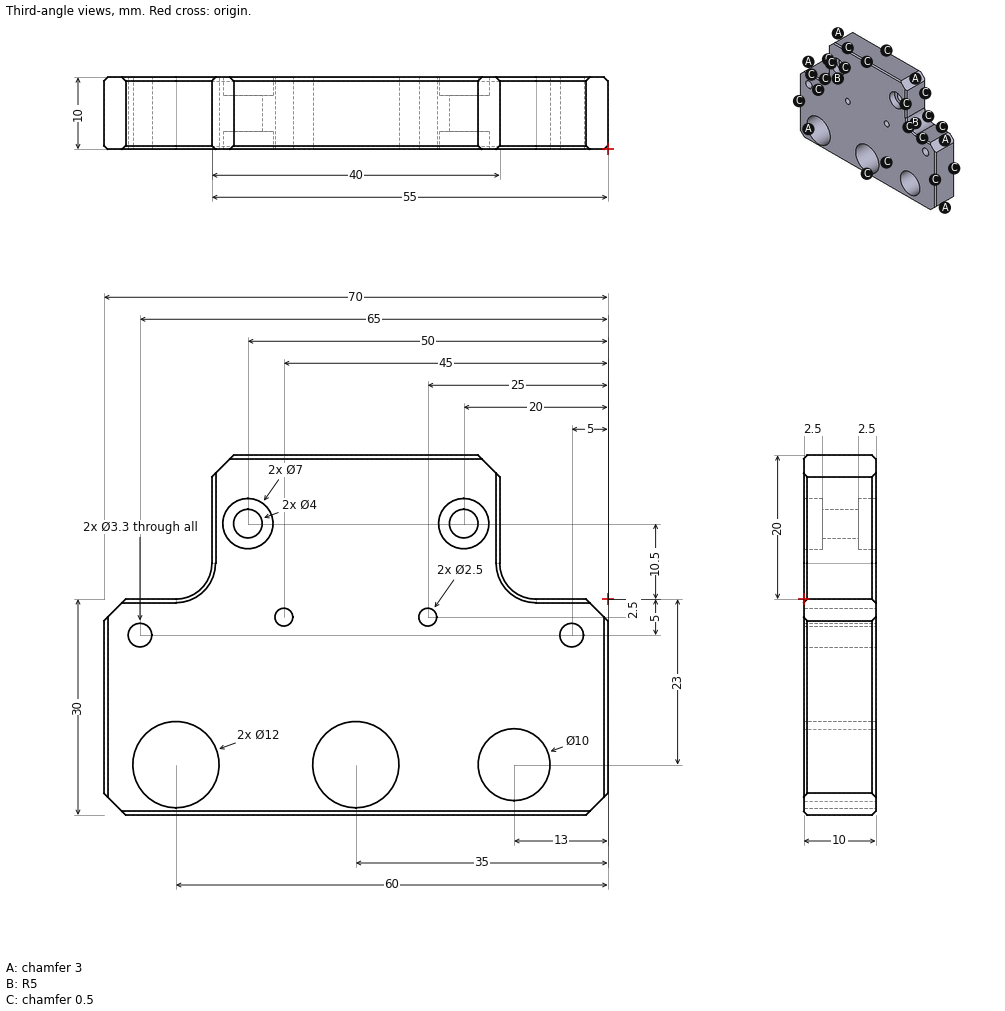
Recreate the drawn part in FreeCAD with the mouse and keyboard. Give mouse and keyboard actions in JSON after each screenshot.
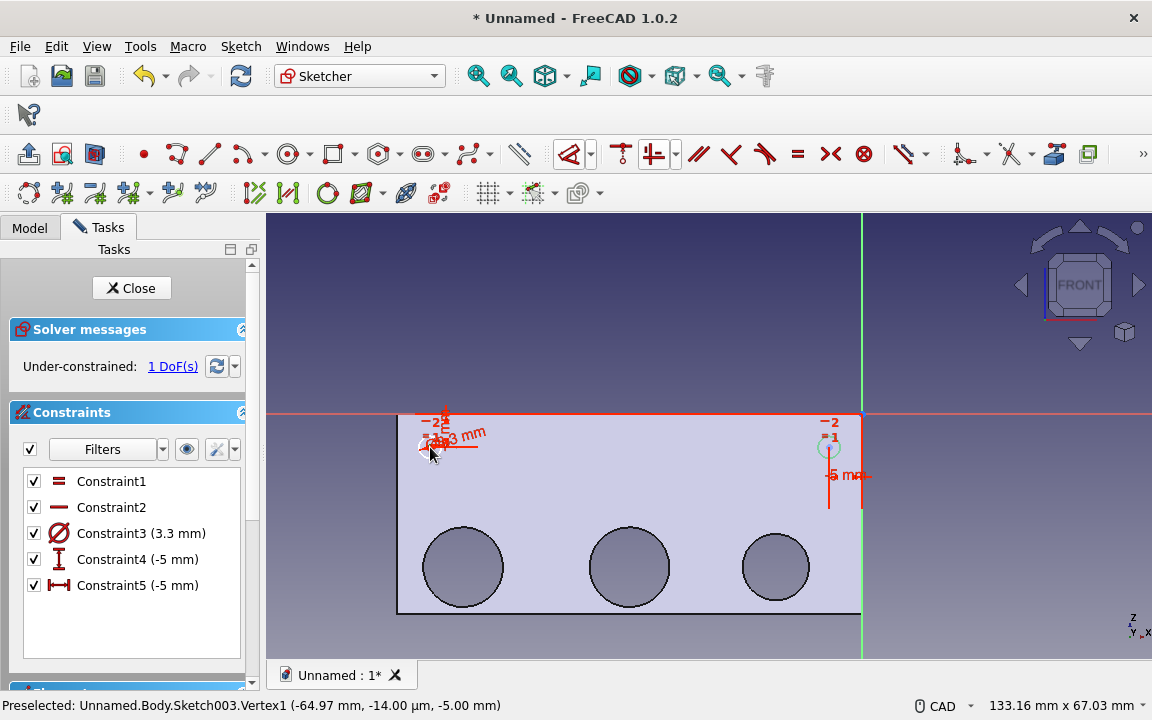
{"action": "left_click", "coordinate": [590, 154]}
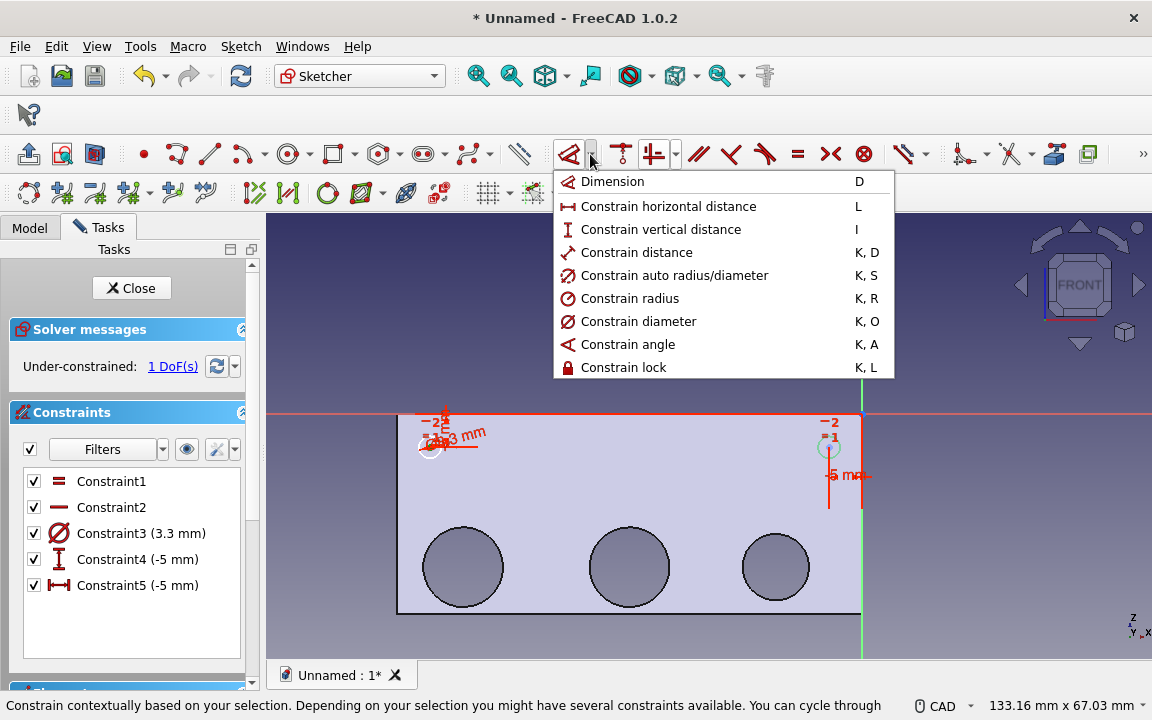
{"action": "left_click", "coordinate": [724, 206]}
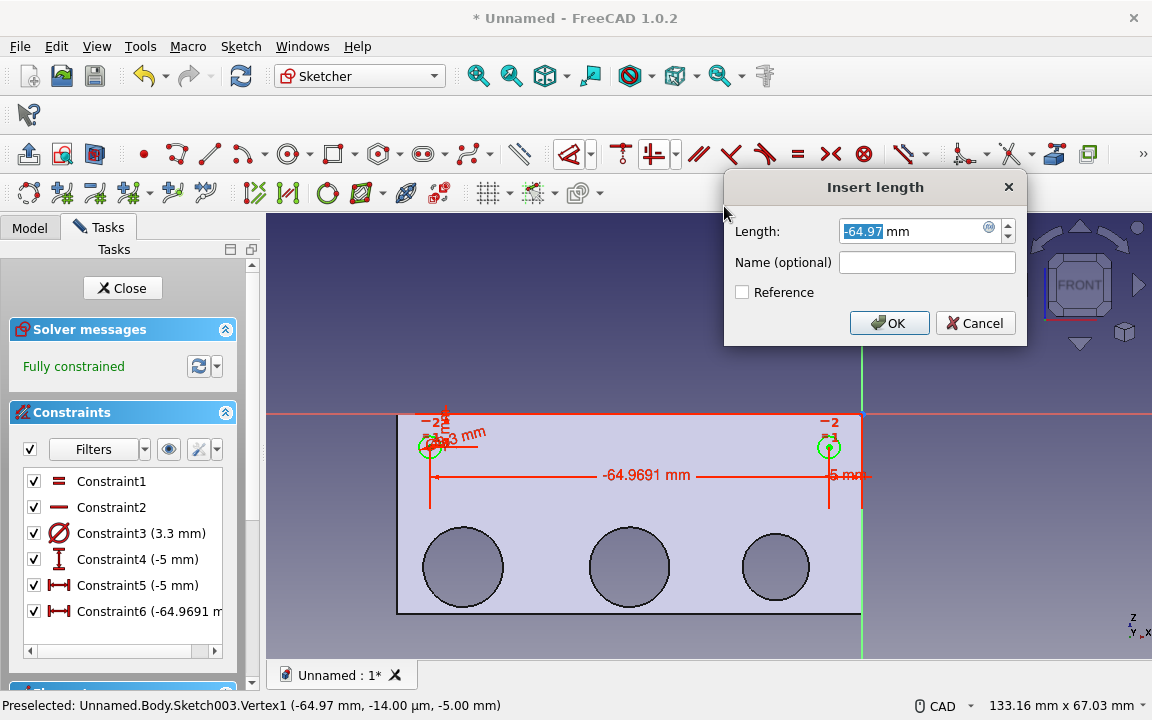
{"action": "type", "text": "-65"}
{"action": "key", "text": "Return"}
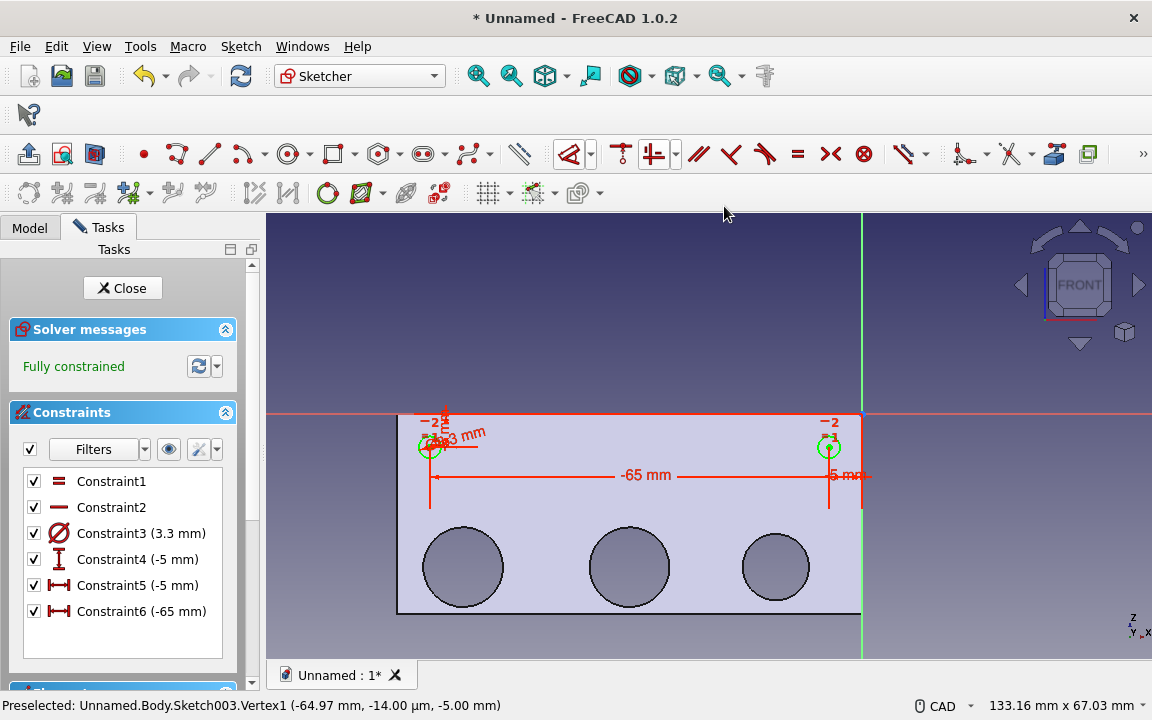
{"action": "left_click", "coordinate": [123, 288]}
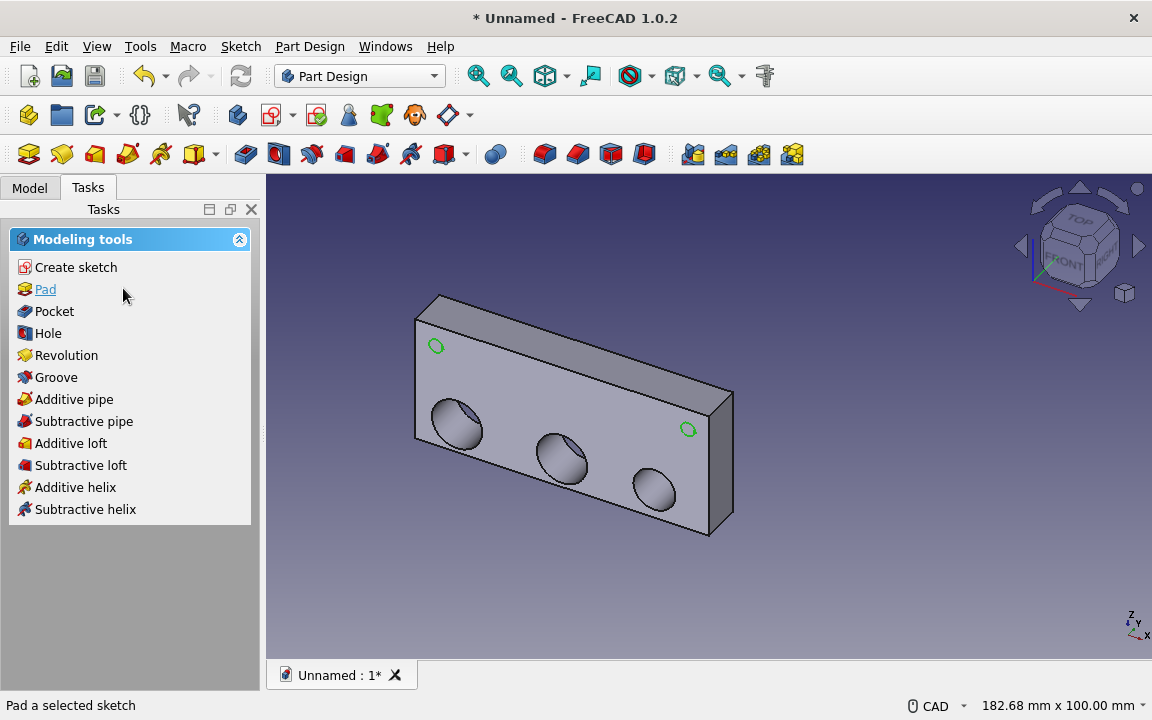
{"action": "left_click", "coordinate": [279, 154]}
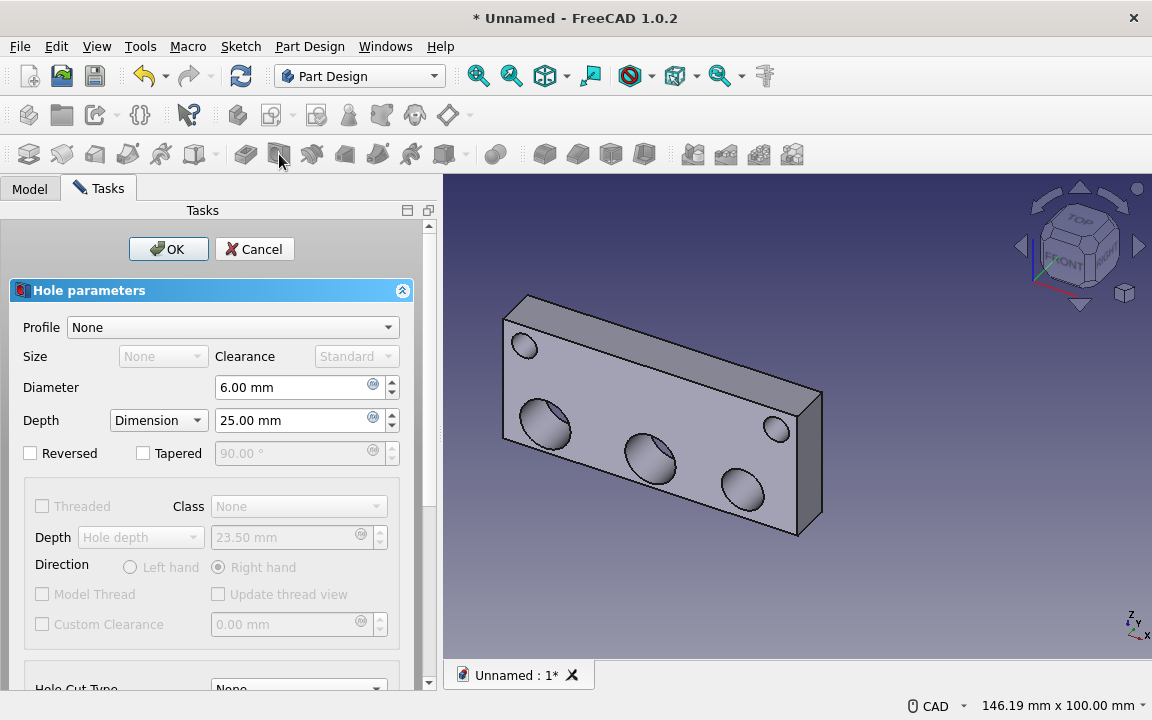
{"action": "triple_click", "coordinate": [300, 388]}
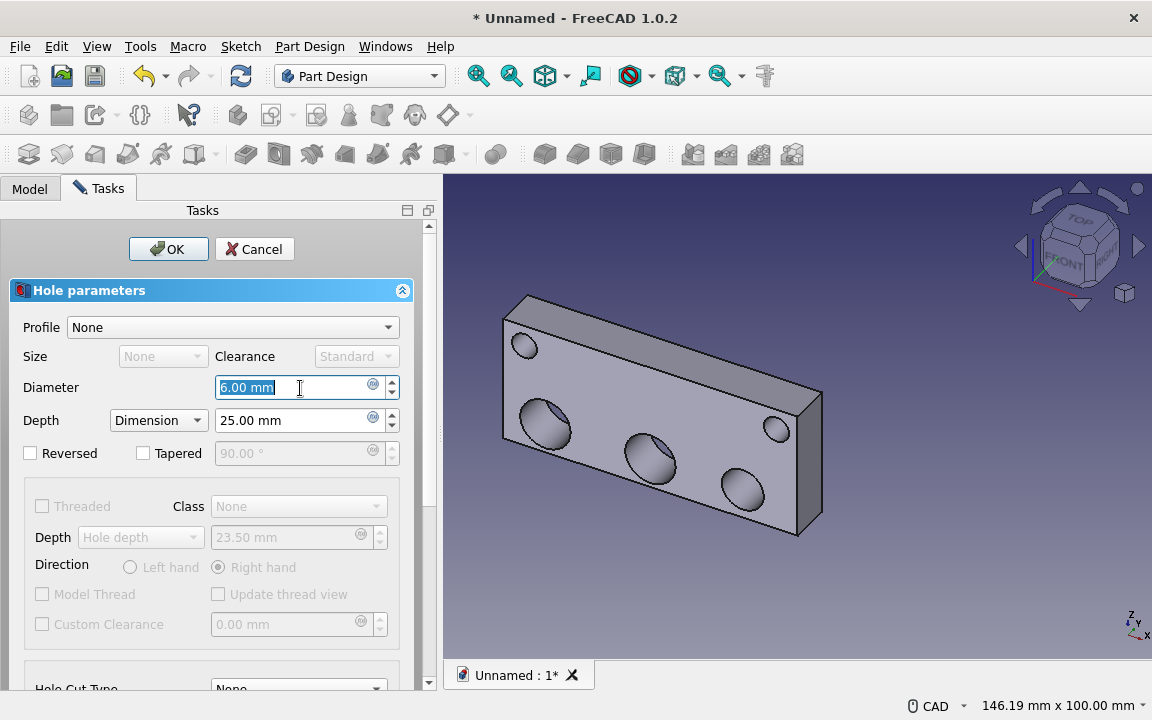
{"action": "type", "text": "3.3"}
{"action": "key", "text": "Tab"}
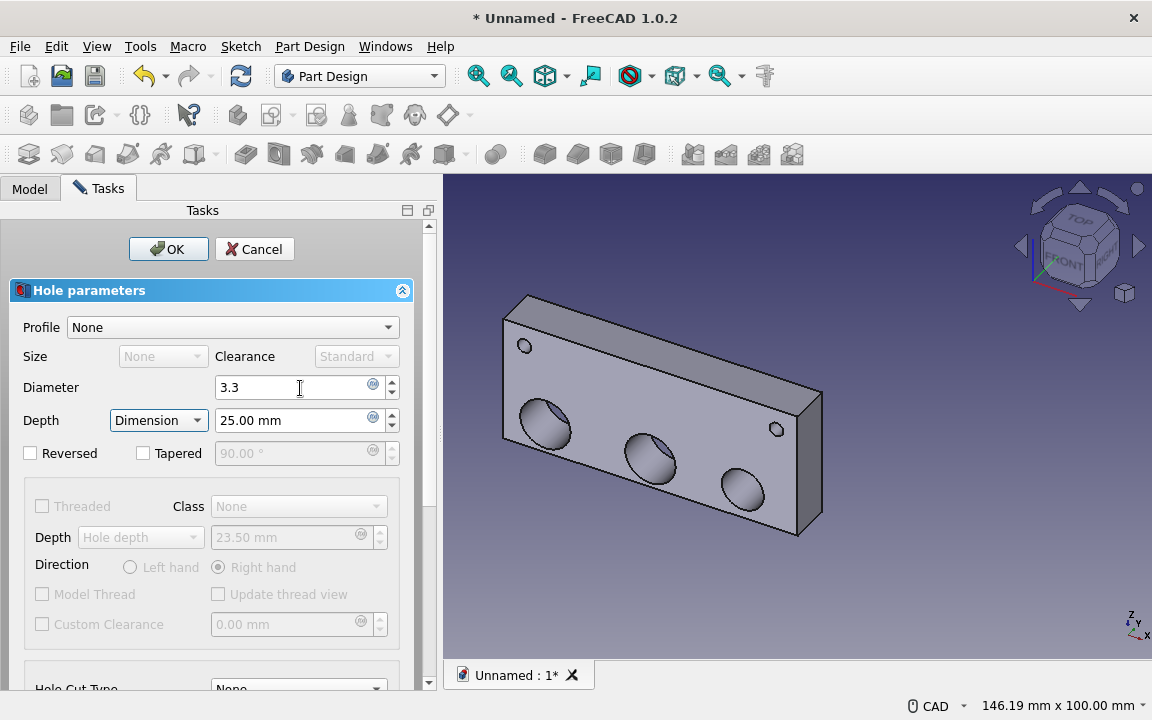
{"action": "left_click", "coordinate": [160, 420]}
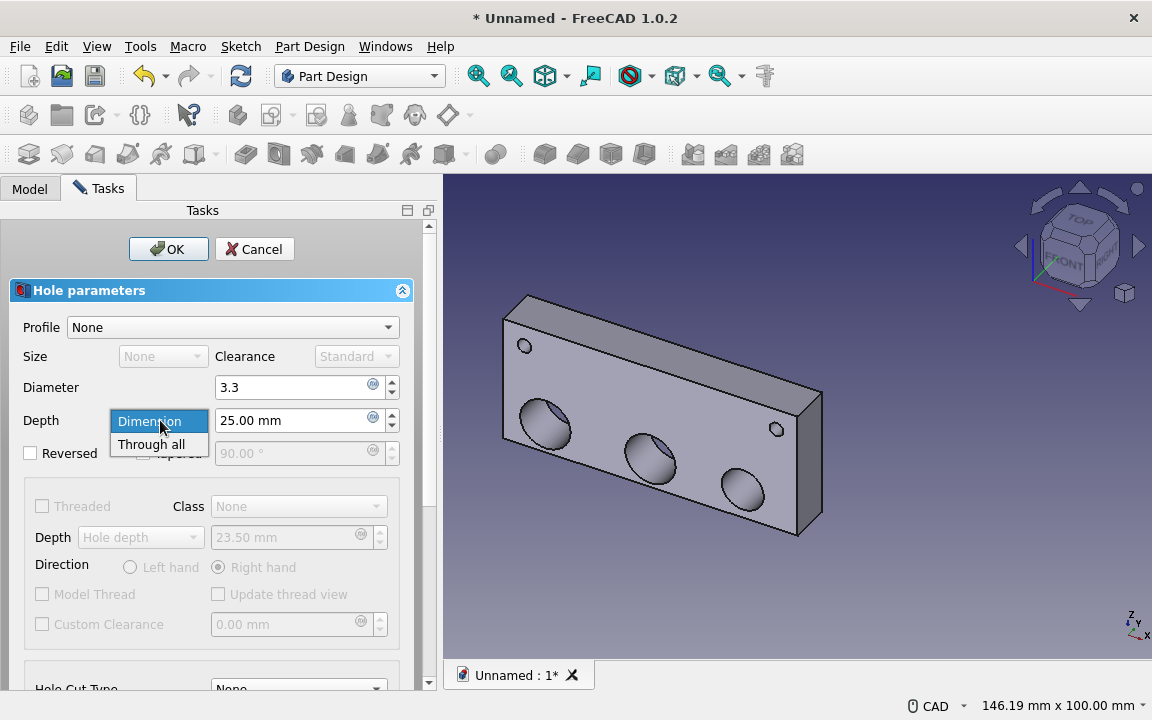
{"action": "left_click", "coordinate": [158, 444]}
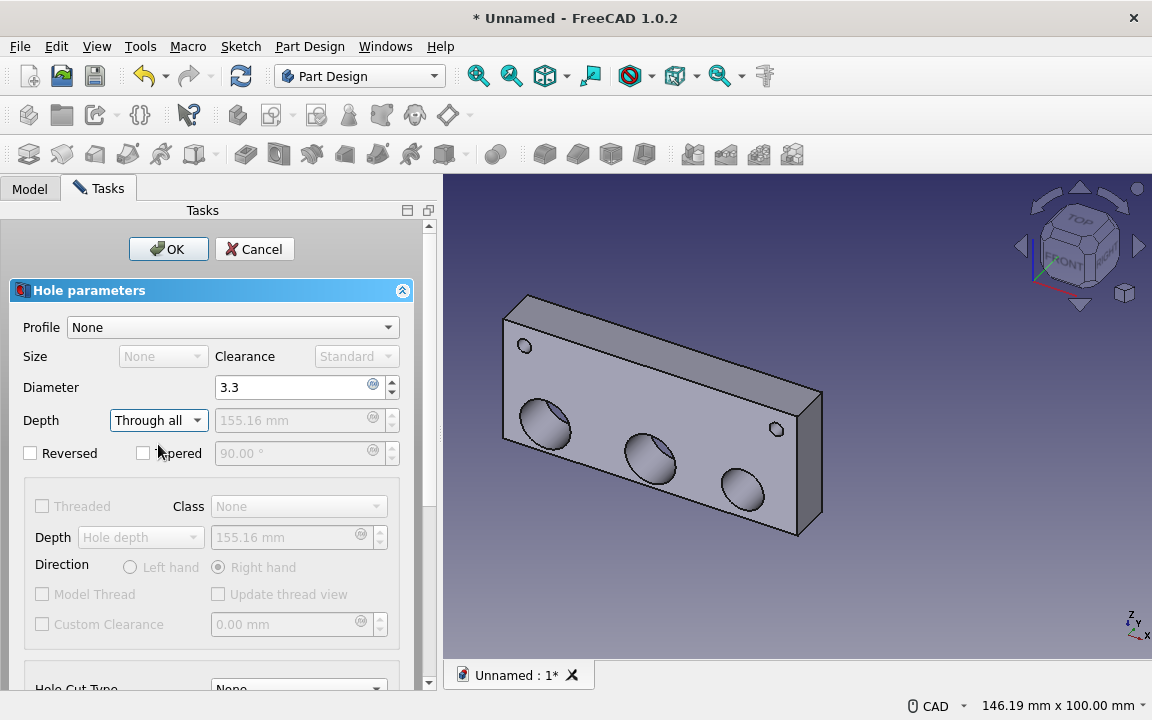
{"action": "left_click", "coordinate": [169, 249]}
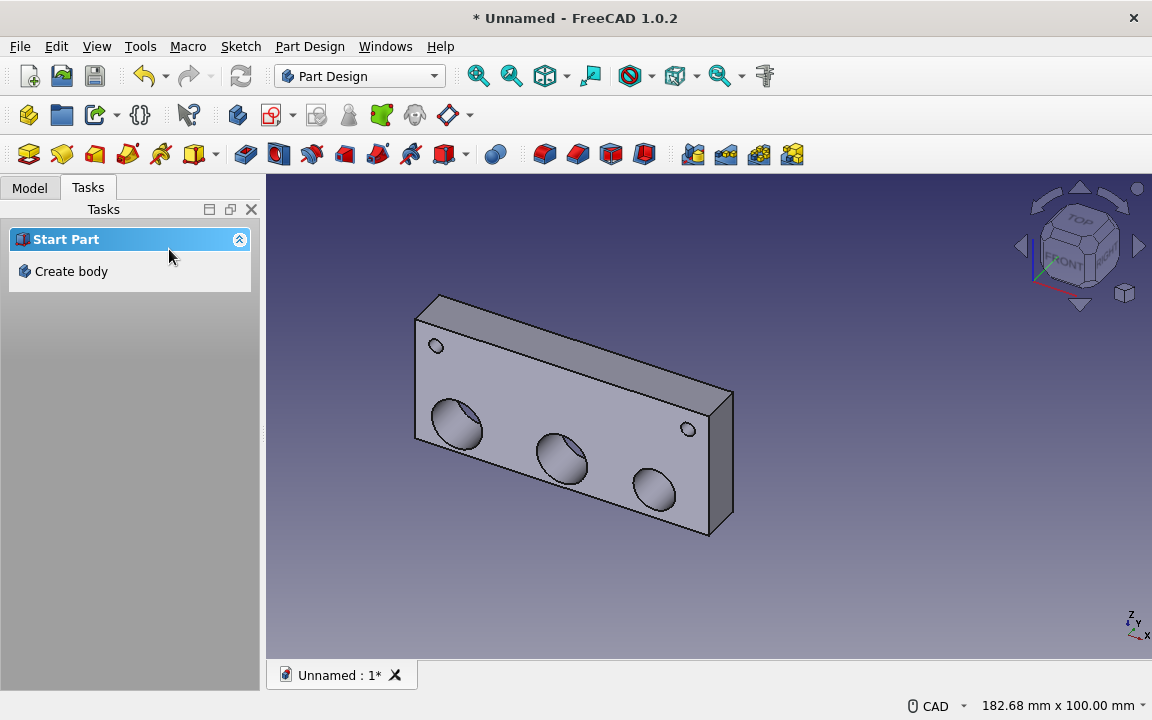
{"action": "left_click", "coordinate": [270, 116]}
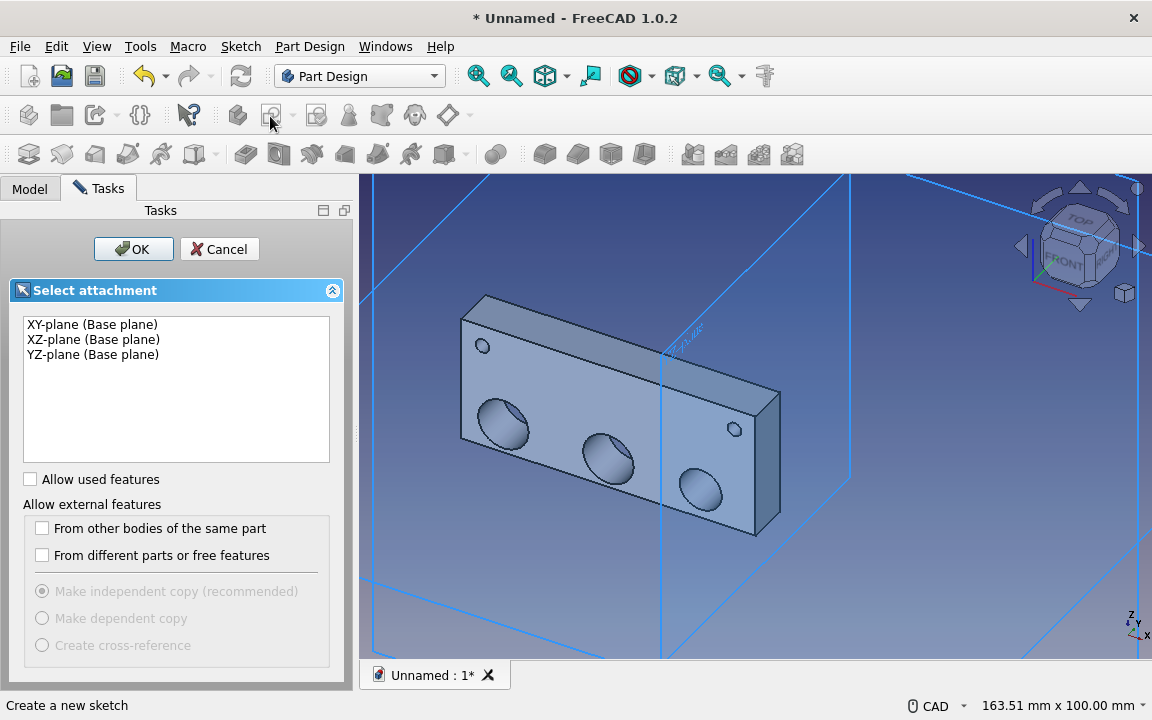
{"action": "left_click", "coordinate": [84, 324]}